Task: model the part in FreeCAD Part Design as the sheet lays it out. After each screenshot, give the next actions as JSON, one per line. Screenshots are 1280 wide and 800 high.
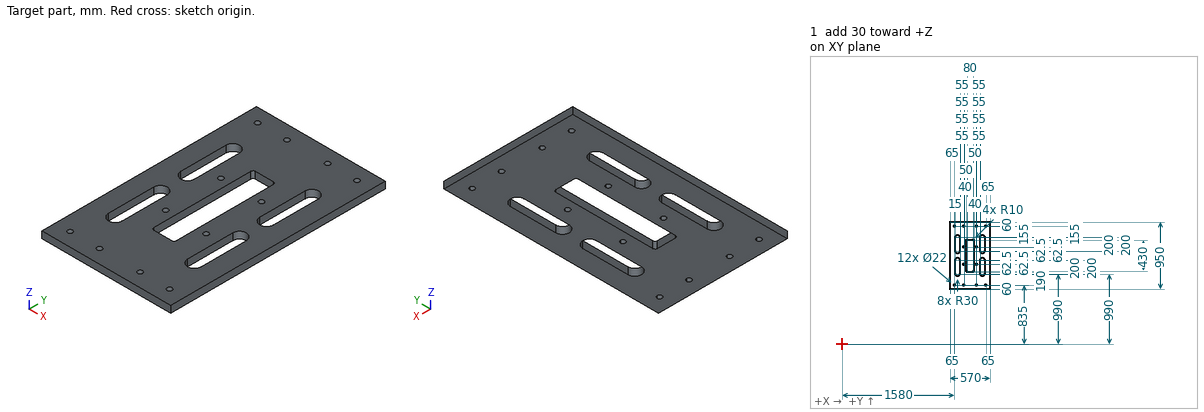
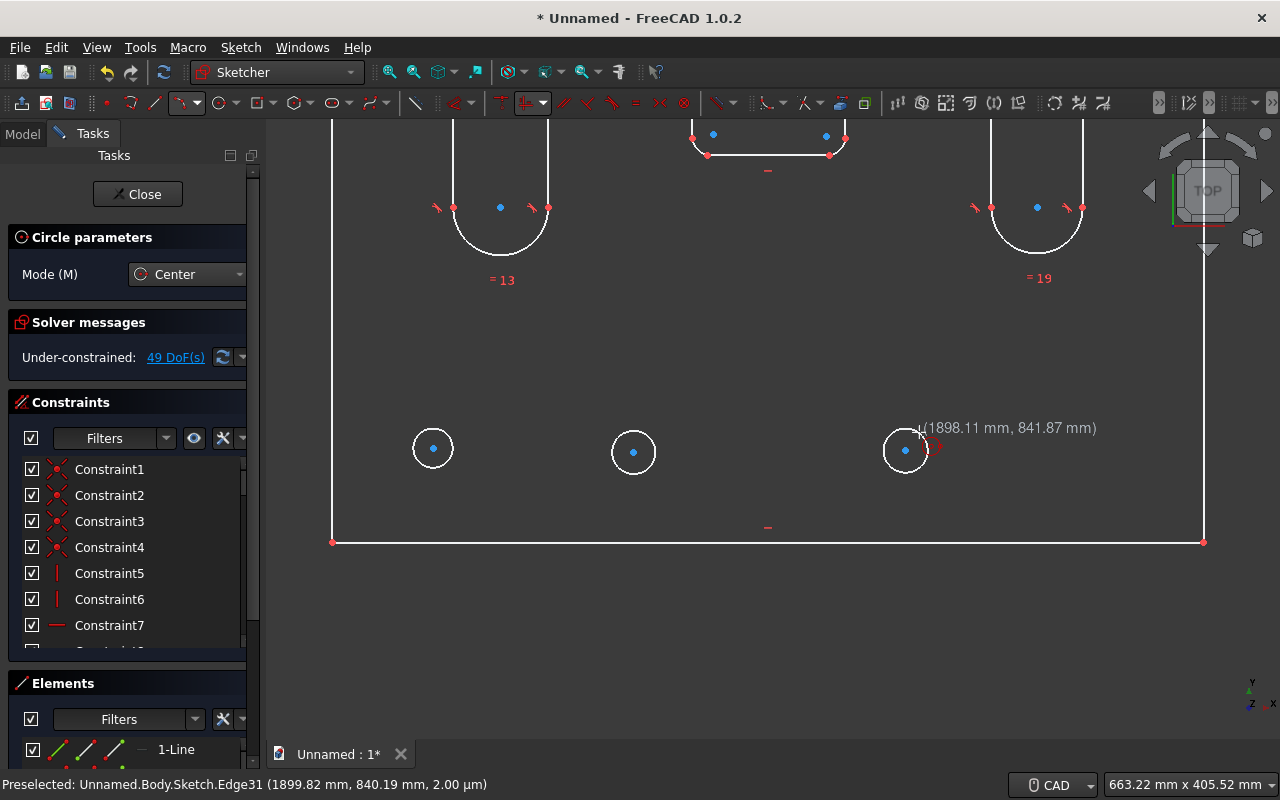
{"action": "scroll", "coordinate": [1105, 443], "scroll_direction": "up", "scroll_amount": 2}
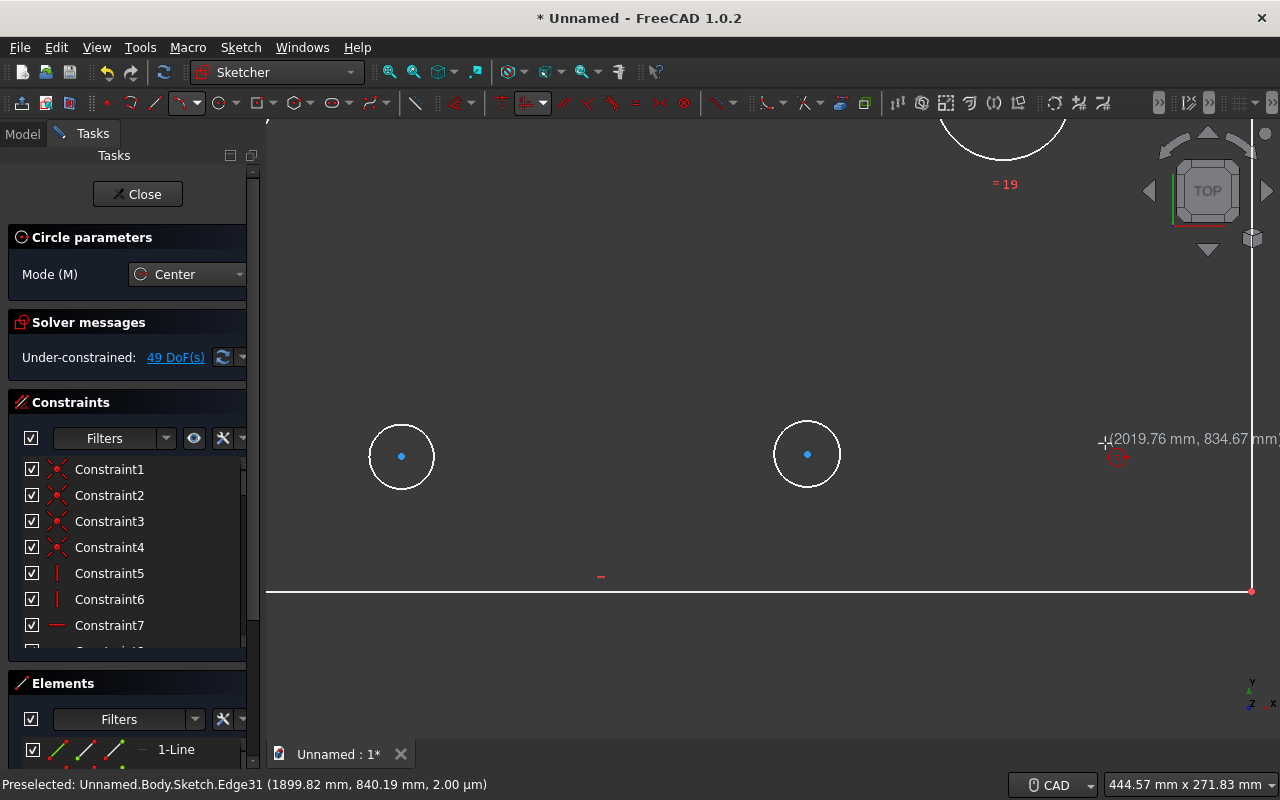
{"action": "scroll", "coordinate": [932, 435], "scroll_direction": "down", "scroll_amount": 11}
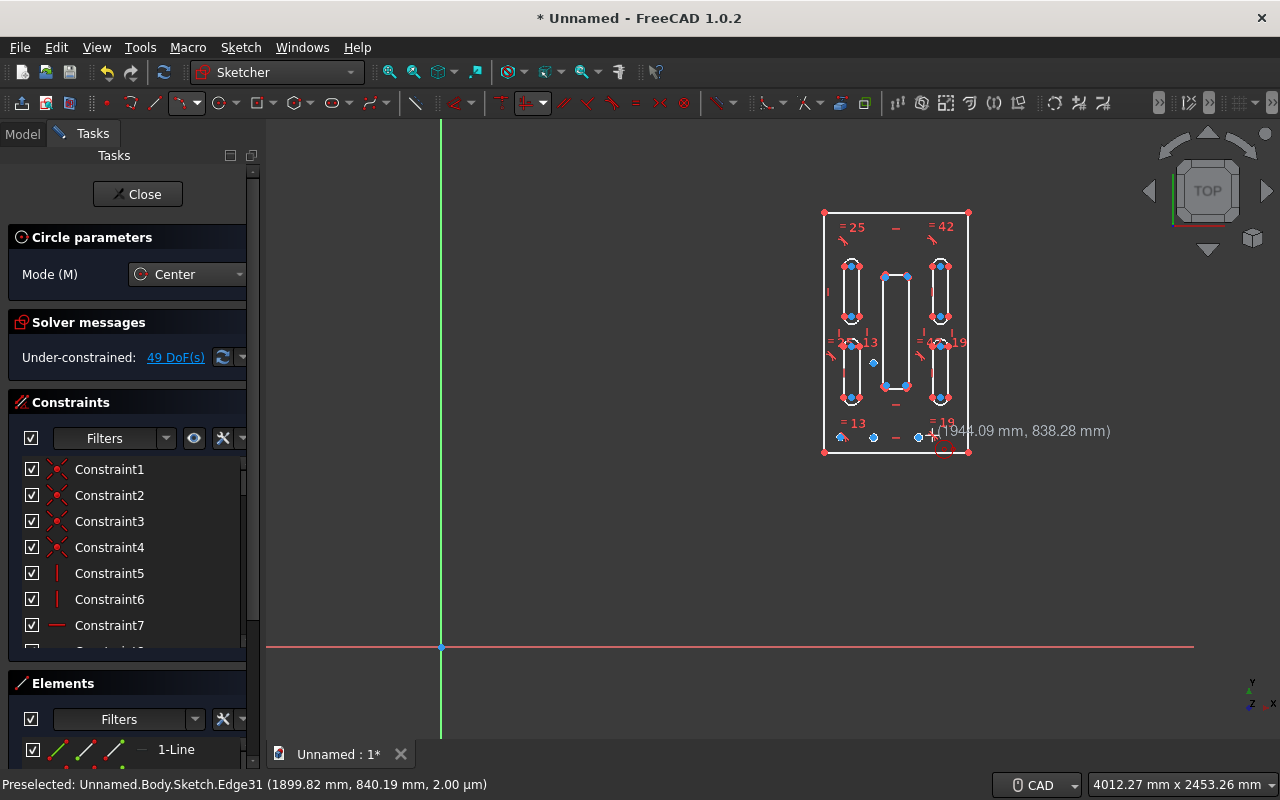
{"action": "left_click", "coordinate": [952, 436]}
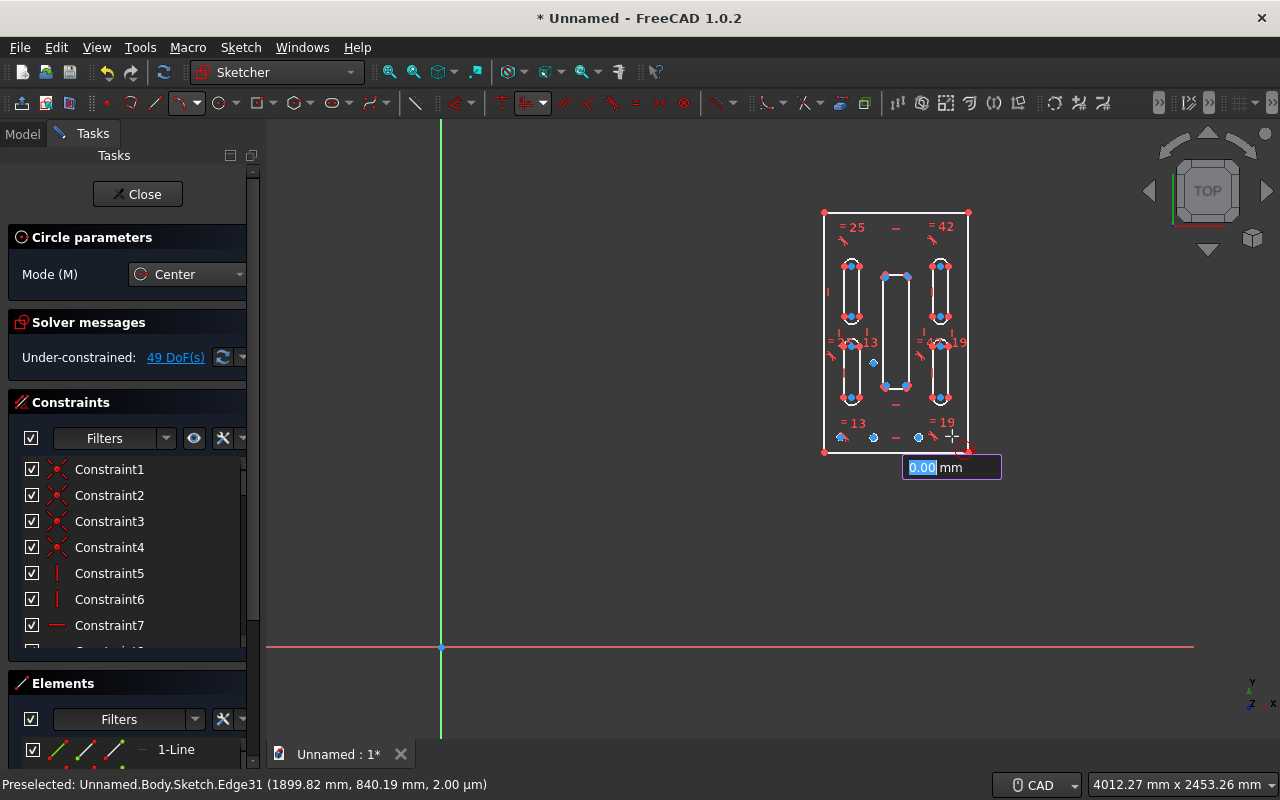
{"action": "scroll", "coordinate": [954, 434], "scroll_direction": "up", "scroll_amount": 9}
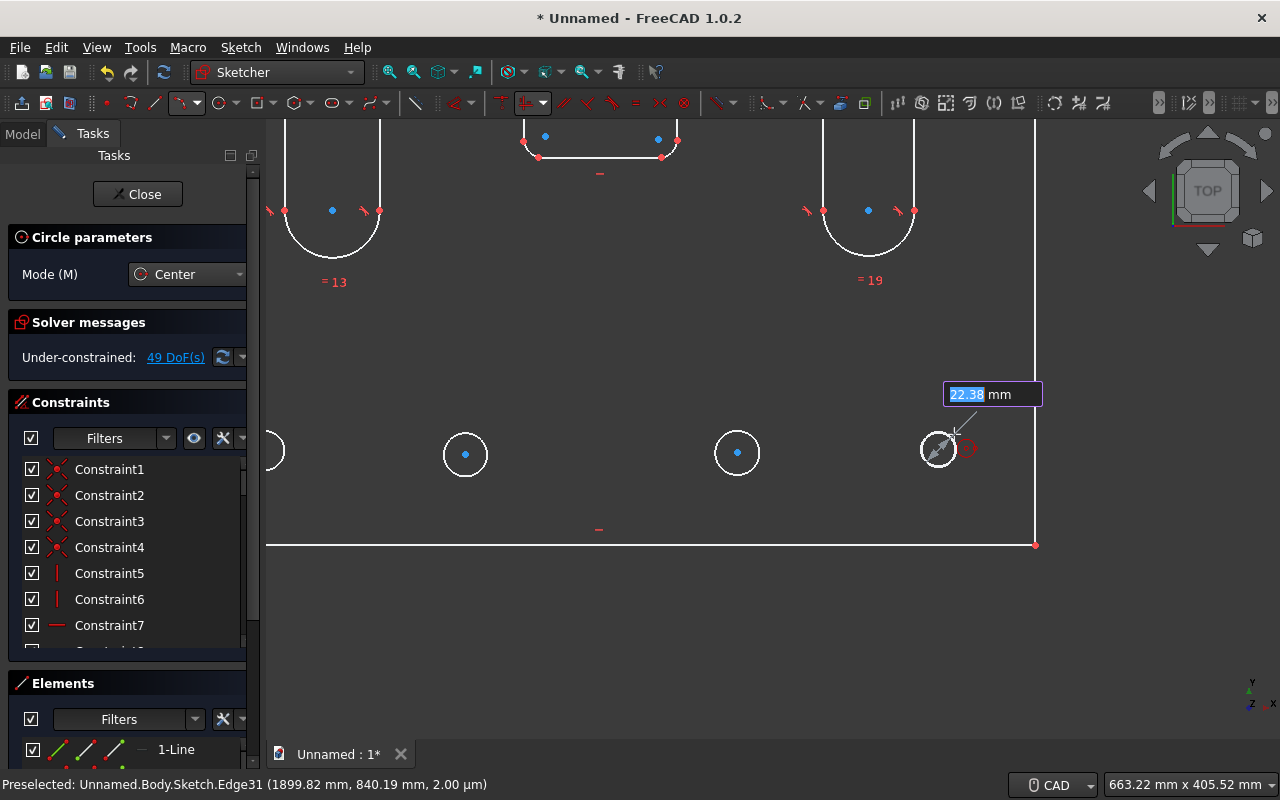
{"action": "left_click", "coordinate": [949, 434]}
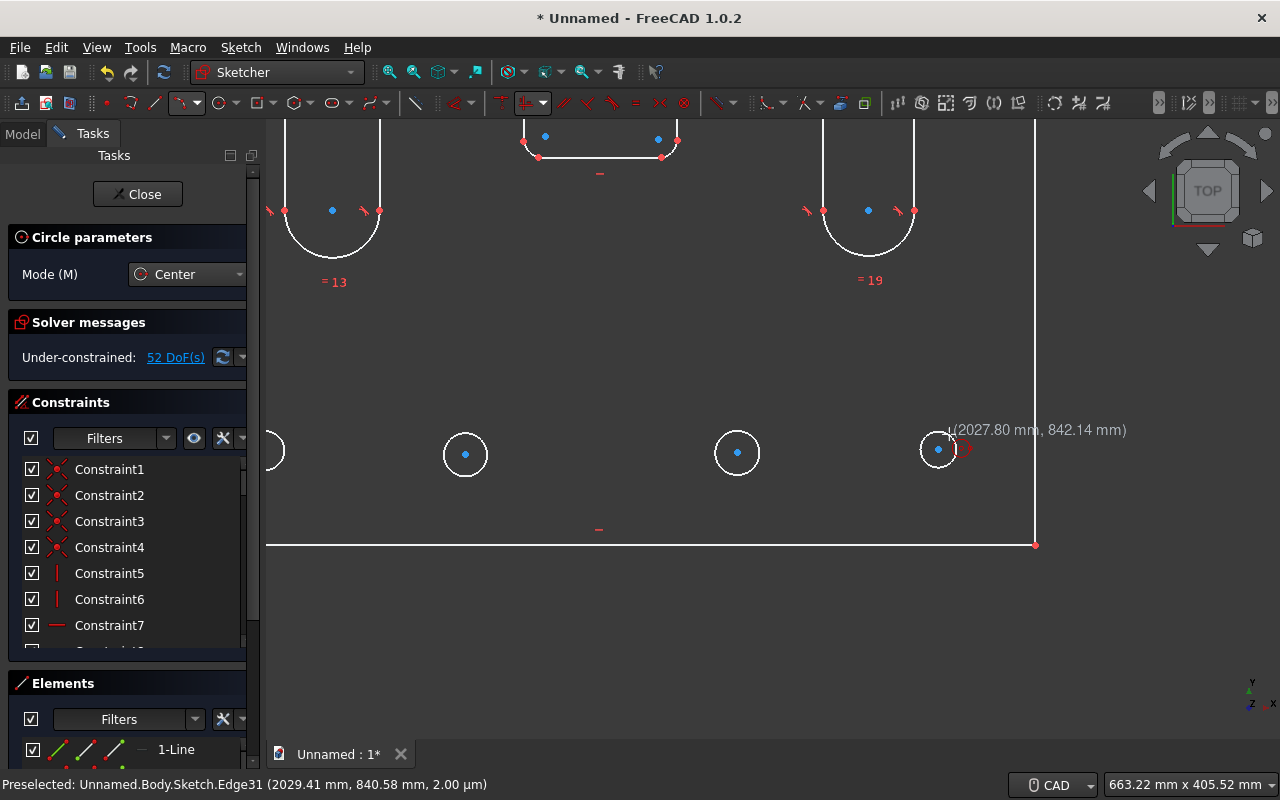
{"action": "scroll", "coordinate": [954, 434], "scroll_direction": "down", "scroll_amount": 9}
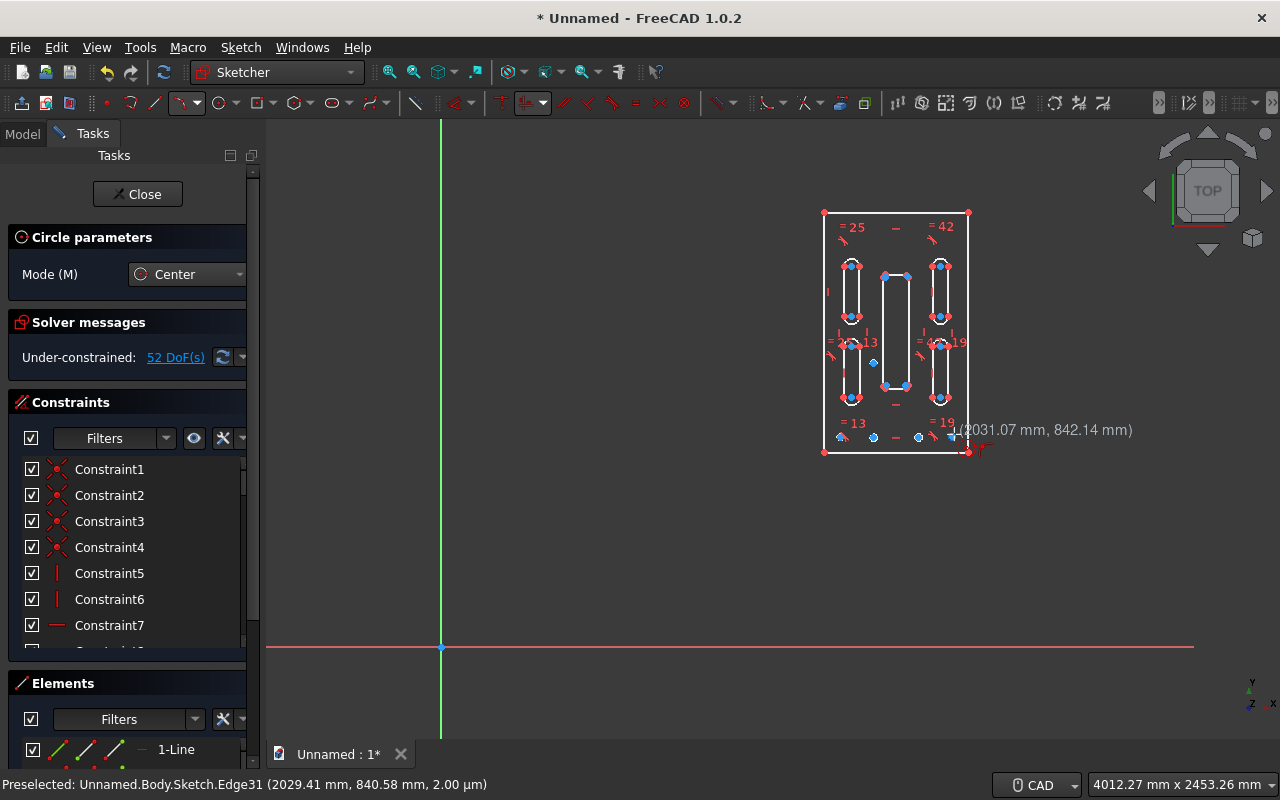
{"action": "scroll", "coordinate": [919, 362], "scroll_direction": "up", "scroll_amount": 11}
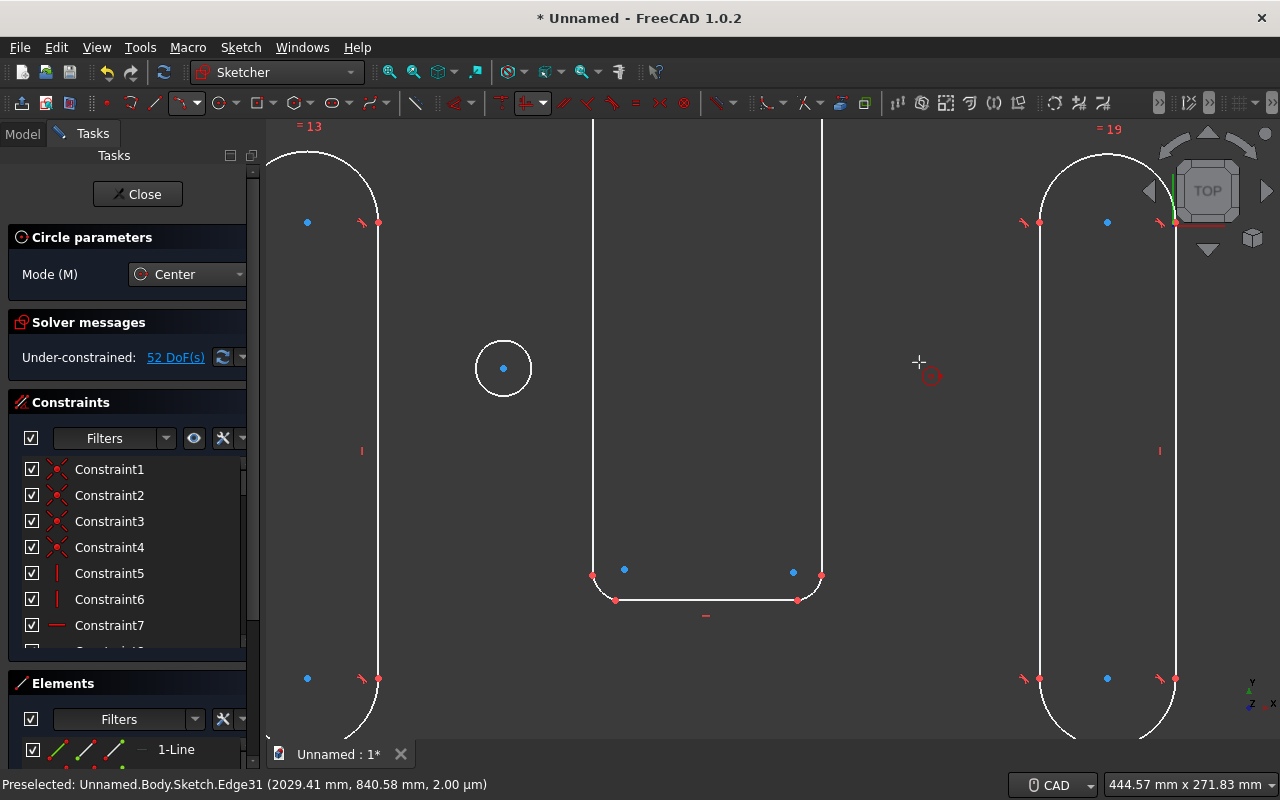
{"action": "scroll", "coordinate": [919, 362], "scroll_direction": "down", "scroll_amount": 11}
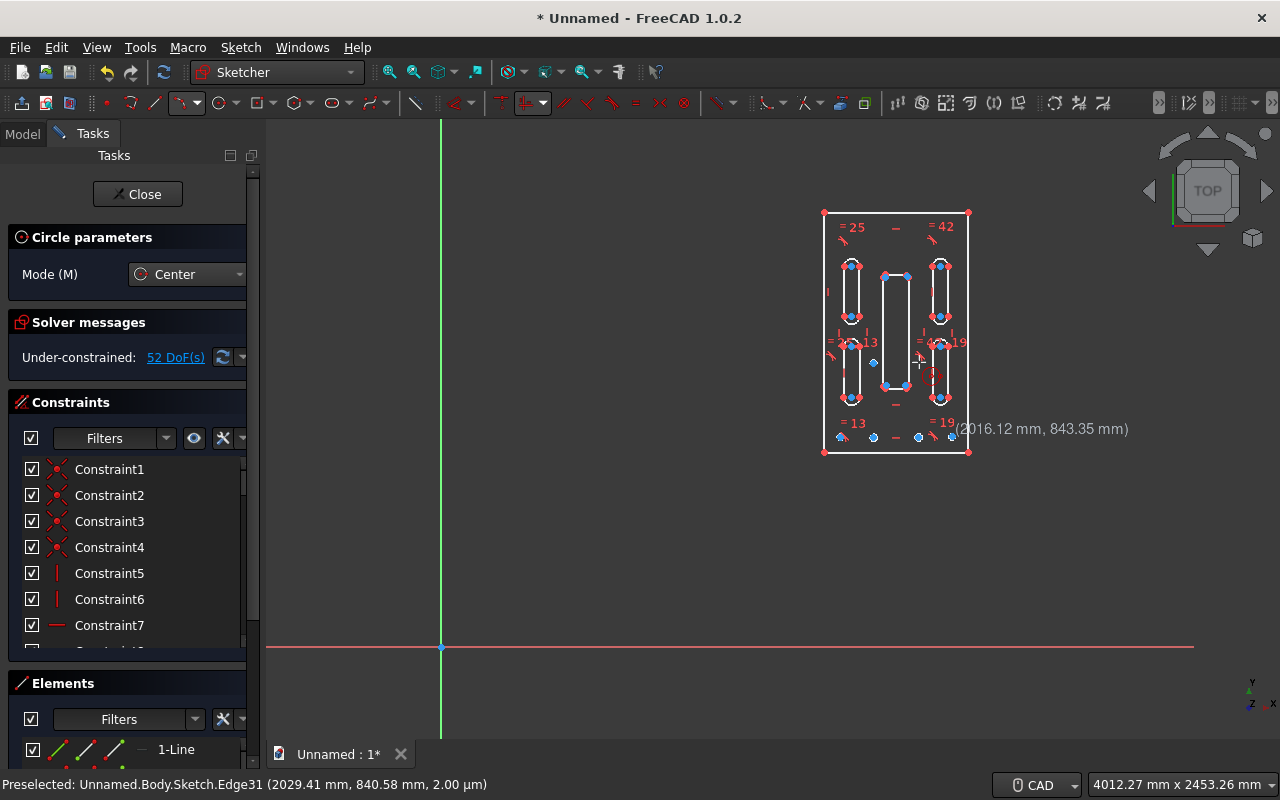
{"action": "scroll", "coordinate": [919, 362], "scroll_direction": "up", "scroll_amount": 3}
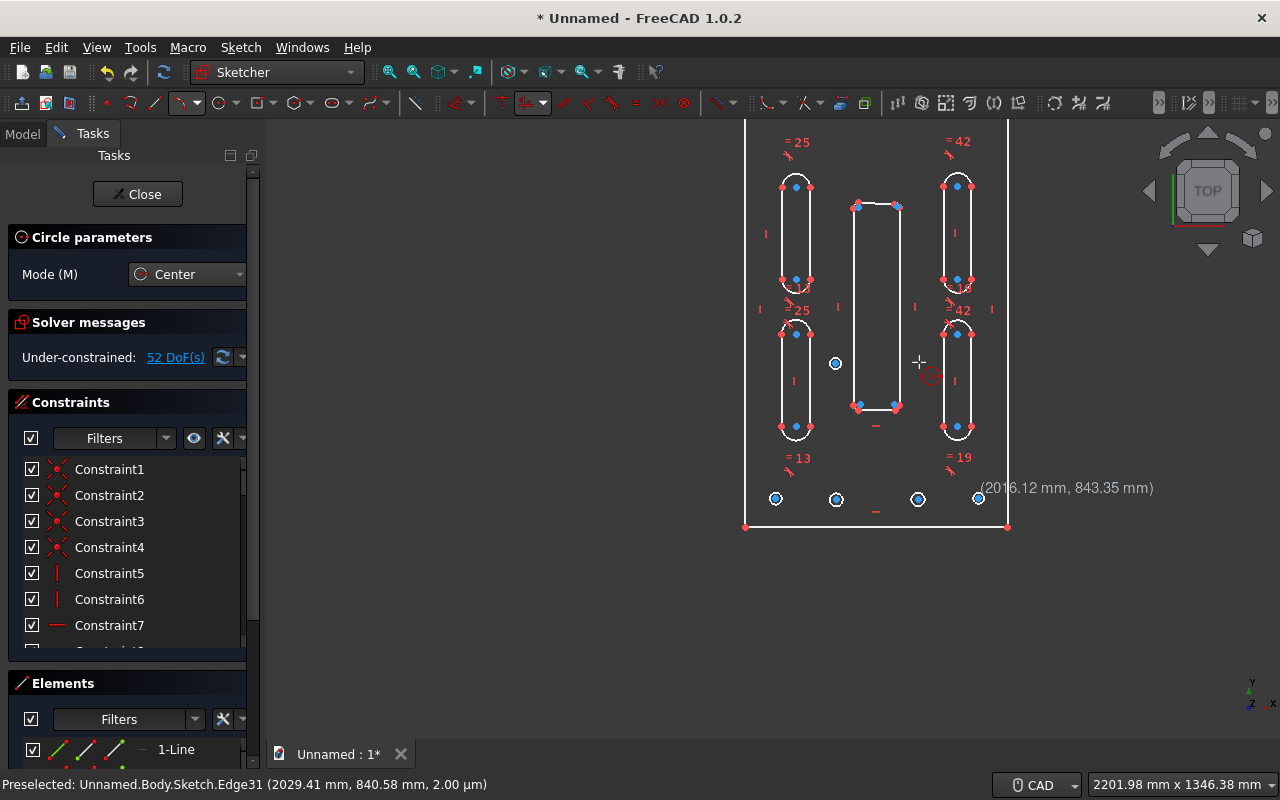
{"action": "left_click", "coordinate": [918, 363]}